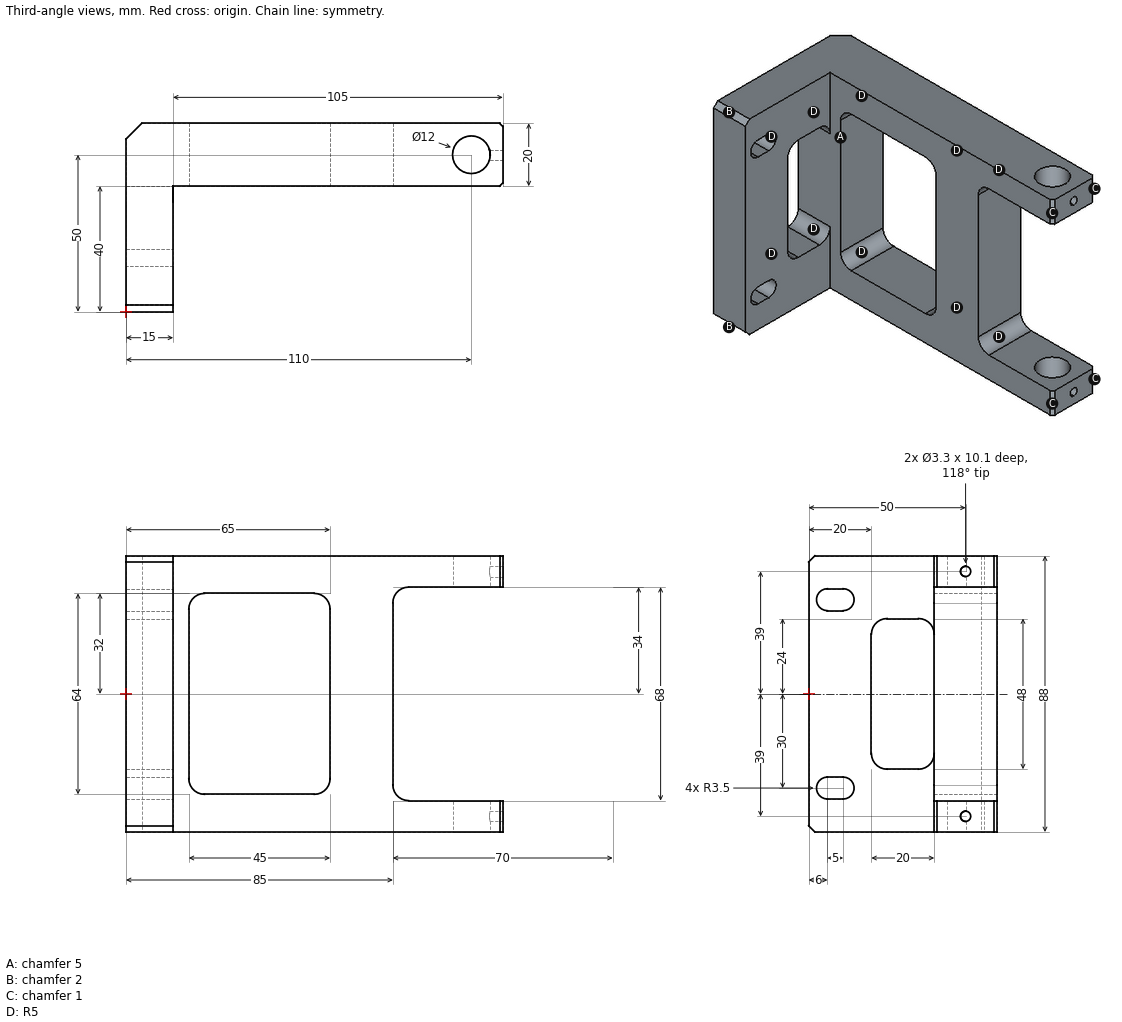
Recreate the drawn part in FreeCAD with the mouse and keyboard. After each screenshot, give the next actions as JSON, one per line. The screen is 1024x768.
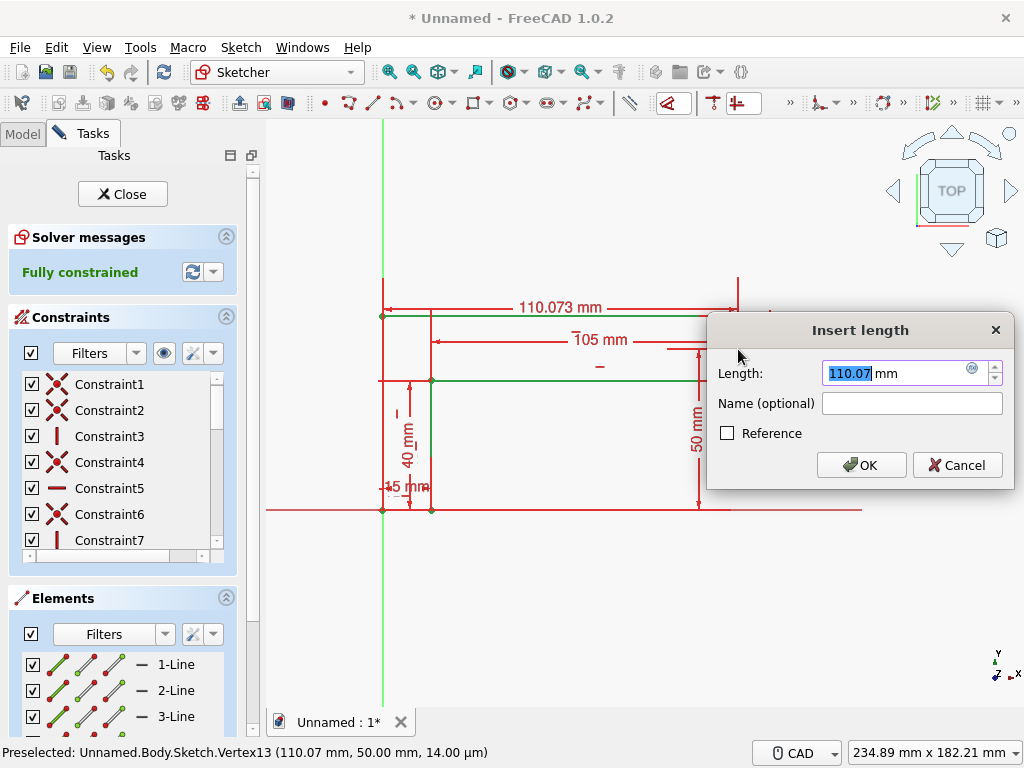
{"action": "type", "text": "110"}
{"action": "key", "text": "Return"}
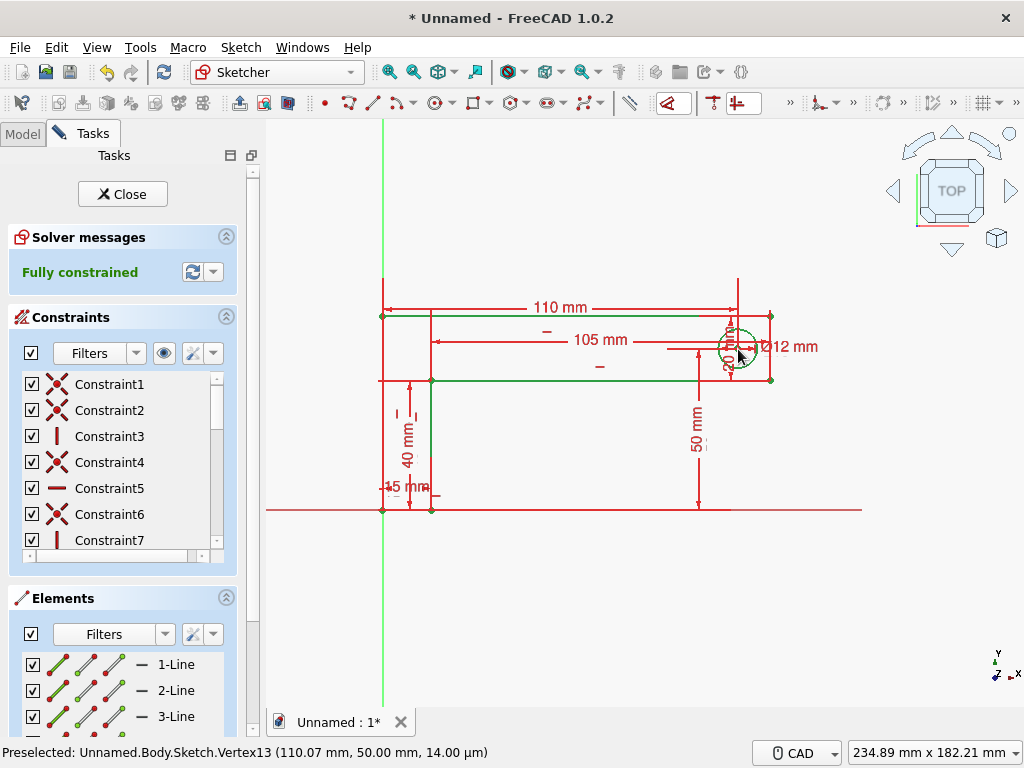
{"action": "left_click", "coordinate": [123, 194]}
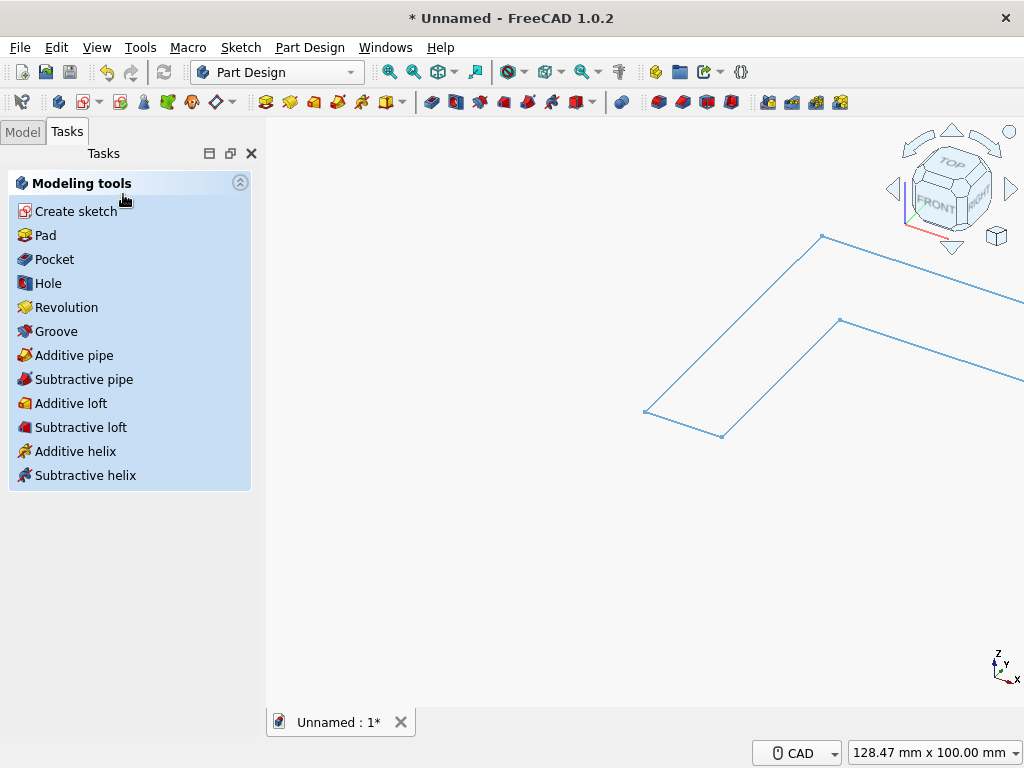
{"action": "left_click", "coordinate": [266, 102]}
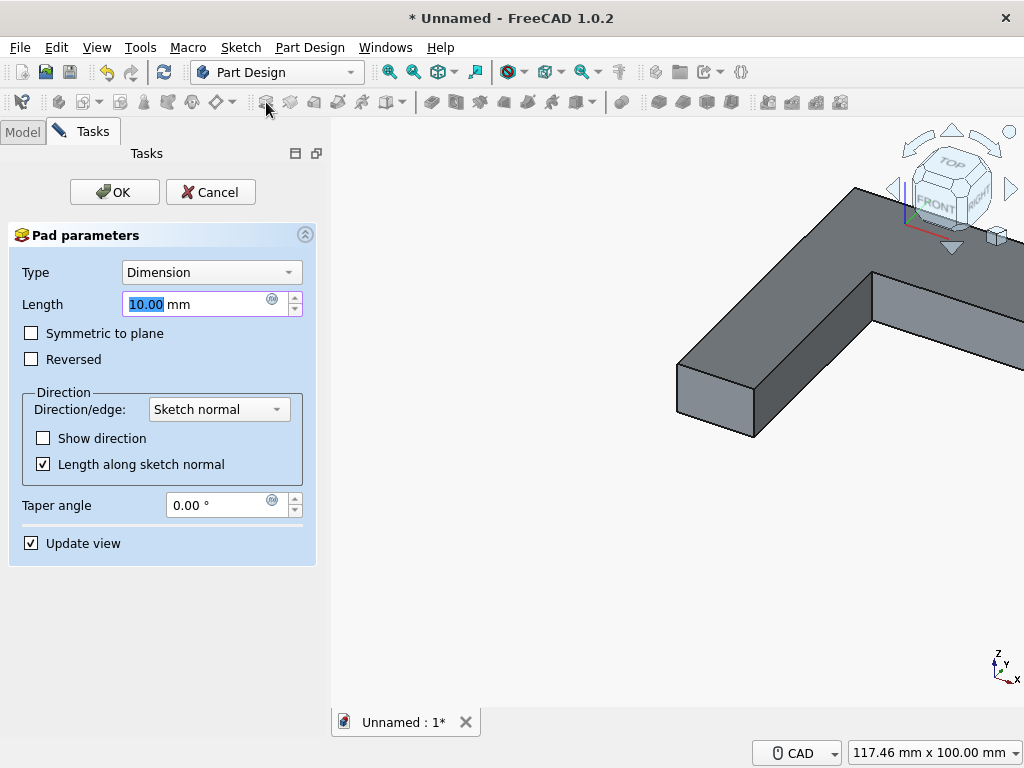
{"action": "type", "text": "88"}
{"action": "key", "text": "Tab"}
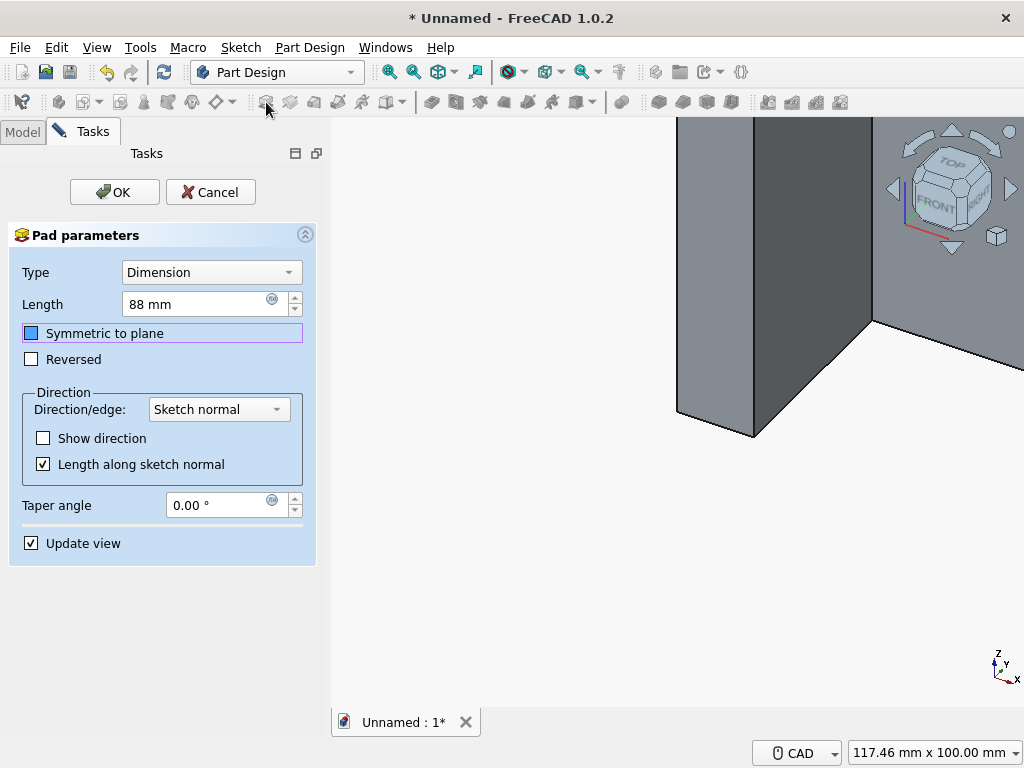
{"action": "left_click", "coordinate": [30, 333]}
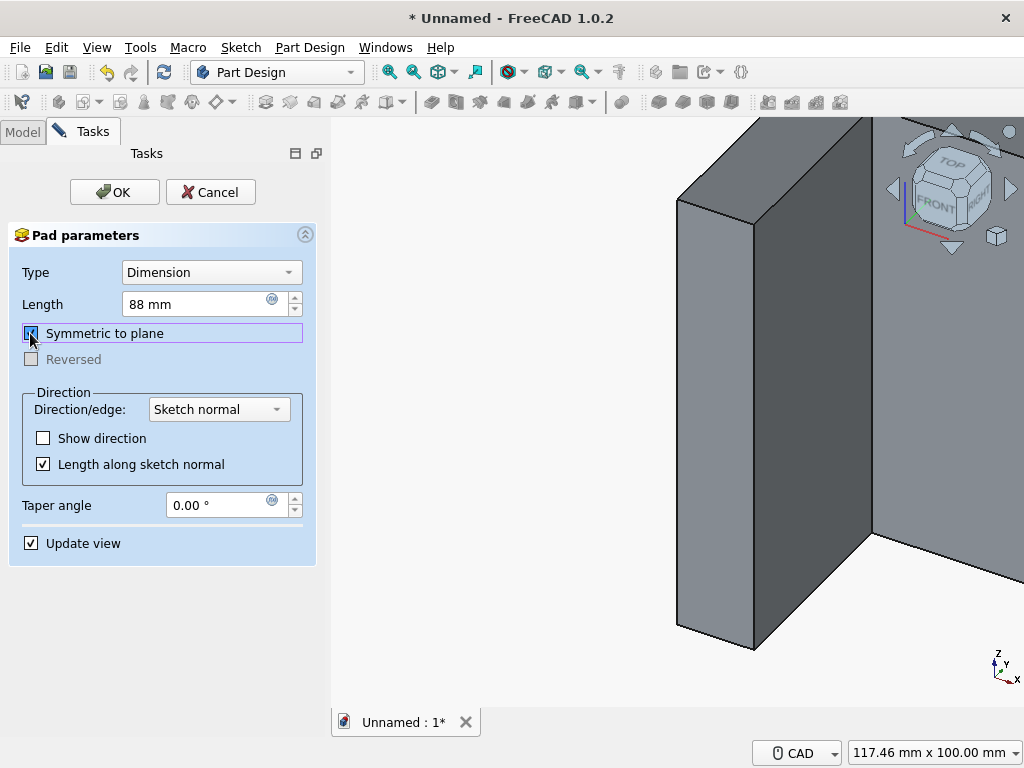
{"action": "left_click", "coordinate": [115, 192]}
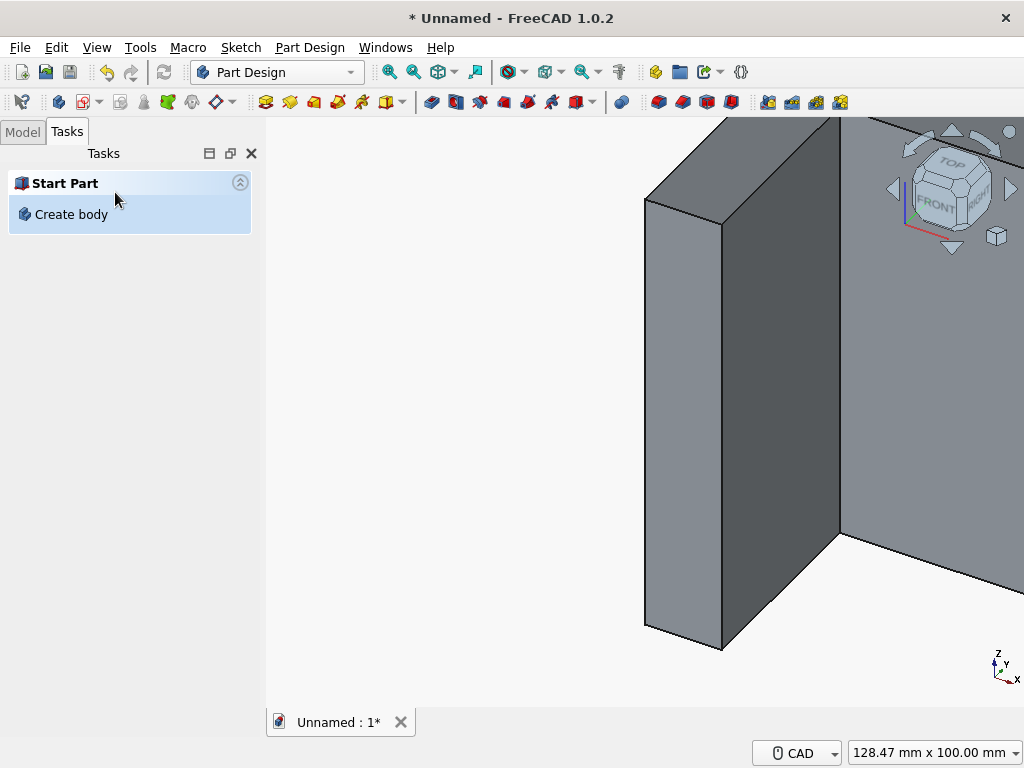
{"action": "left_click", "coordinate": [390, 72]}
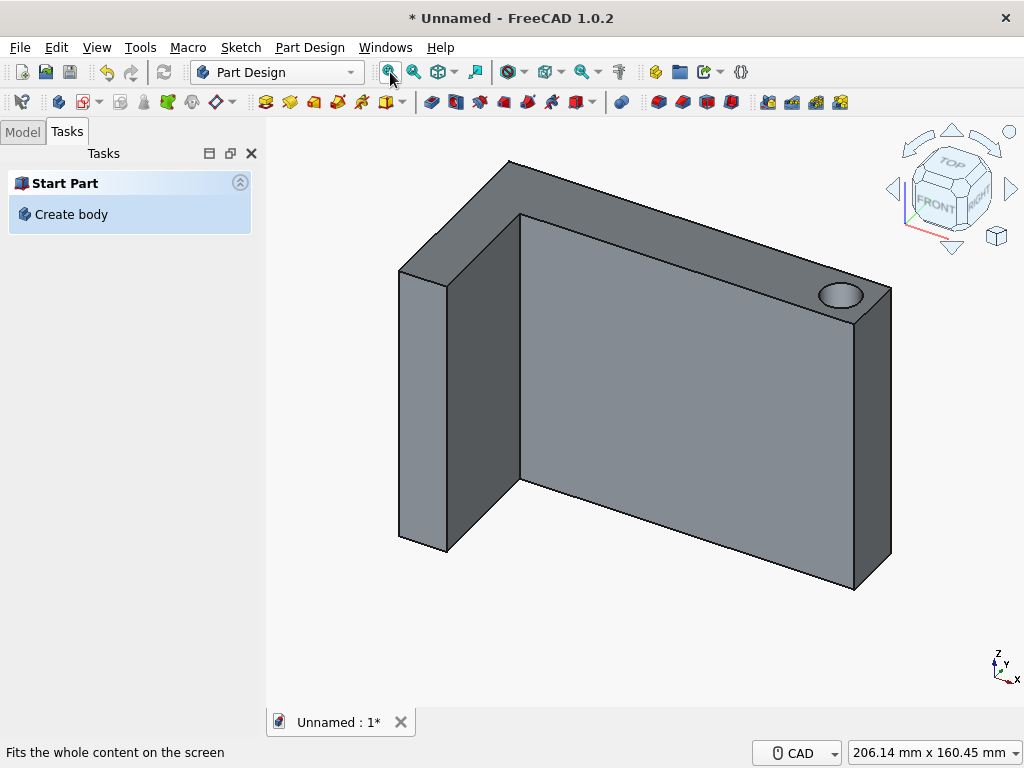
{"action": "key", "text": "4"}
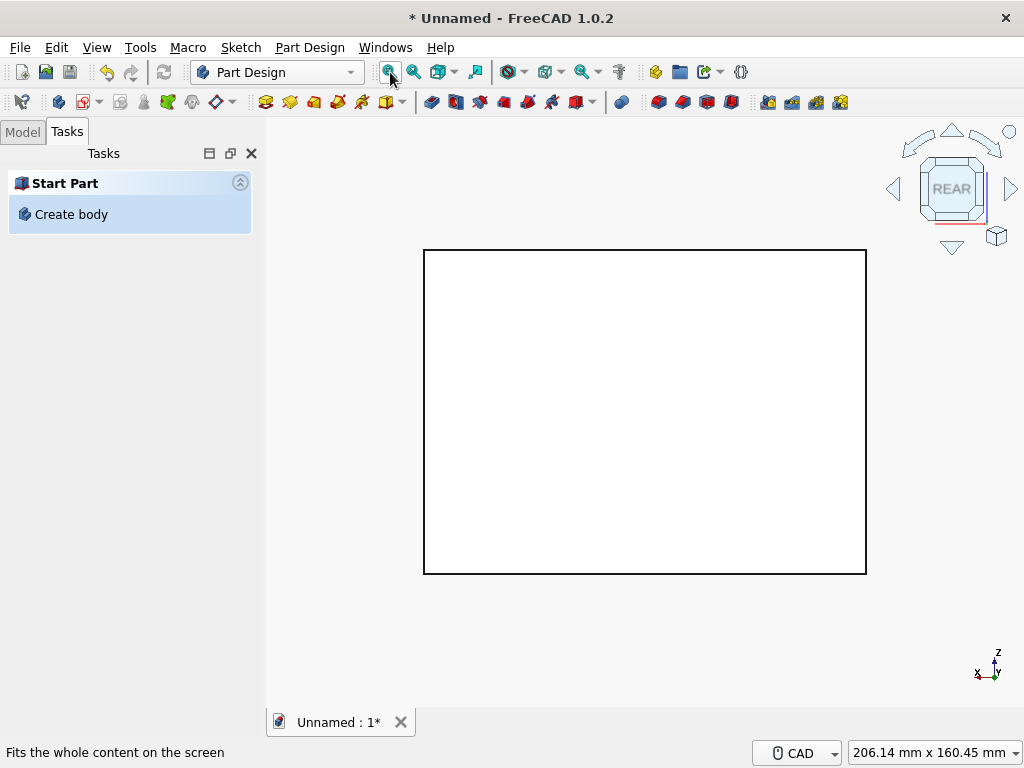
{"action": "left_click", "coordinate": [645, 411]}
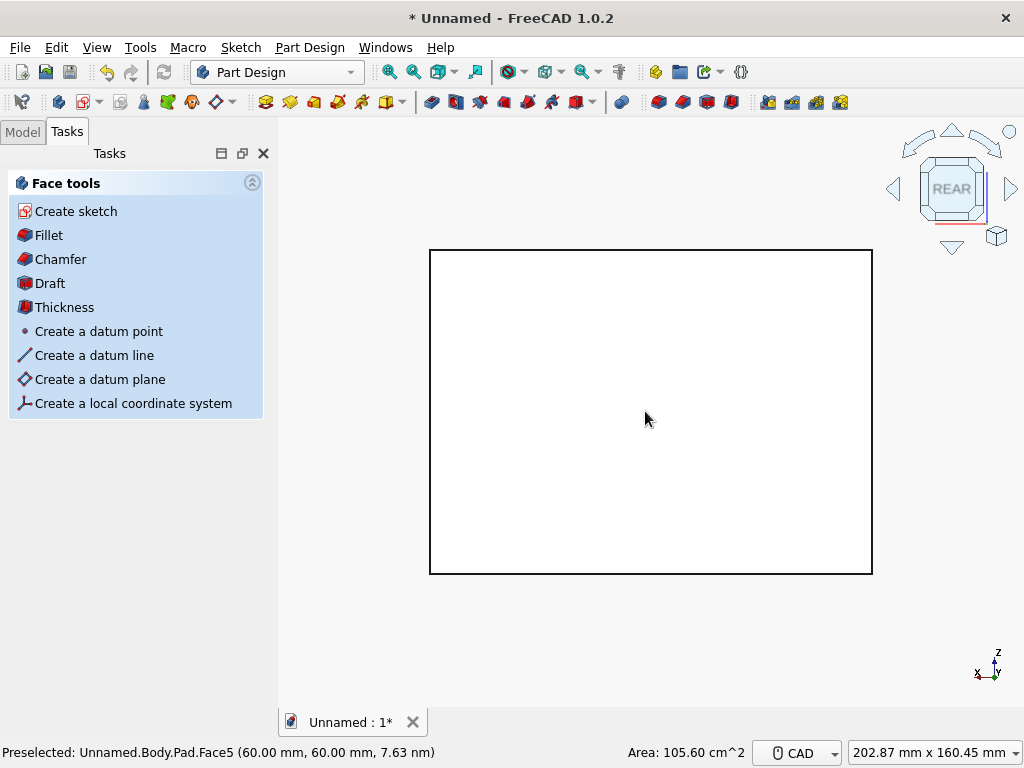
{"action": "left_click", "coordinate": [84, 102]}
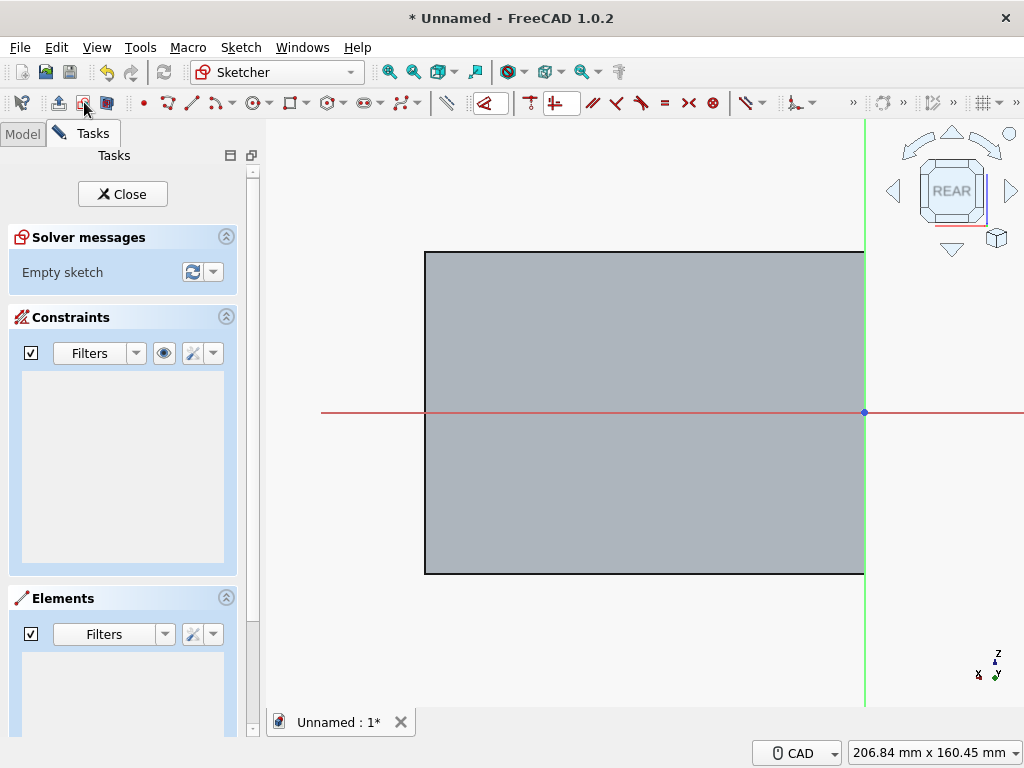
{"action": "scroll", "coordinate": [568, 413], "scroll_direction": "down", "scroll_amount": 2}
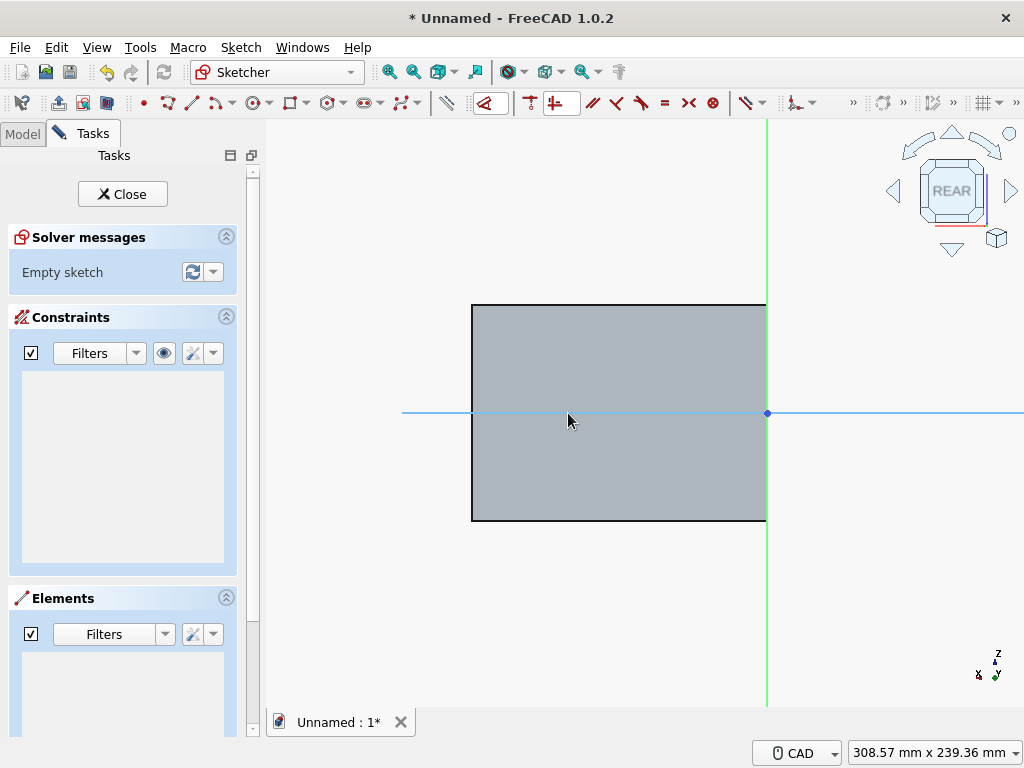
{"action": "key", "text": "g r"}